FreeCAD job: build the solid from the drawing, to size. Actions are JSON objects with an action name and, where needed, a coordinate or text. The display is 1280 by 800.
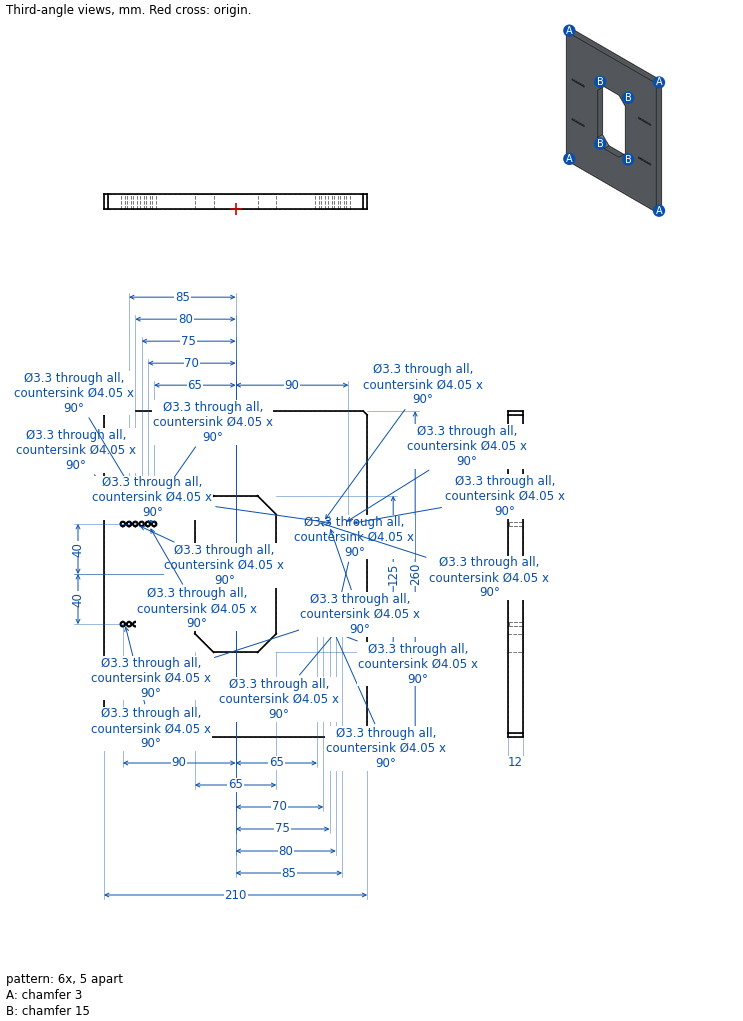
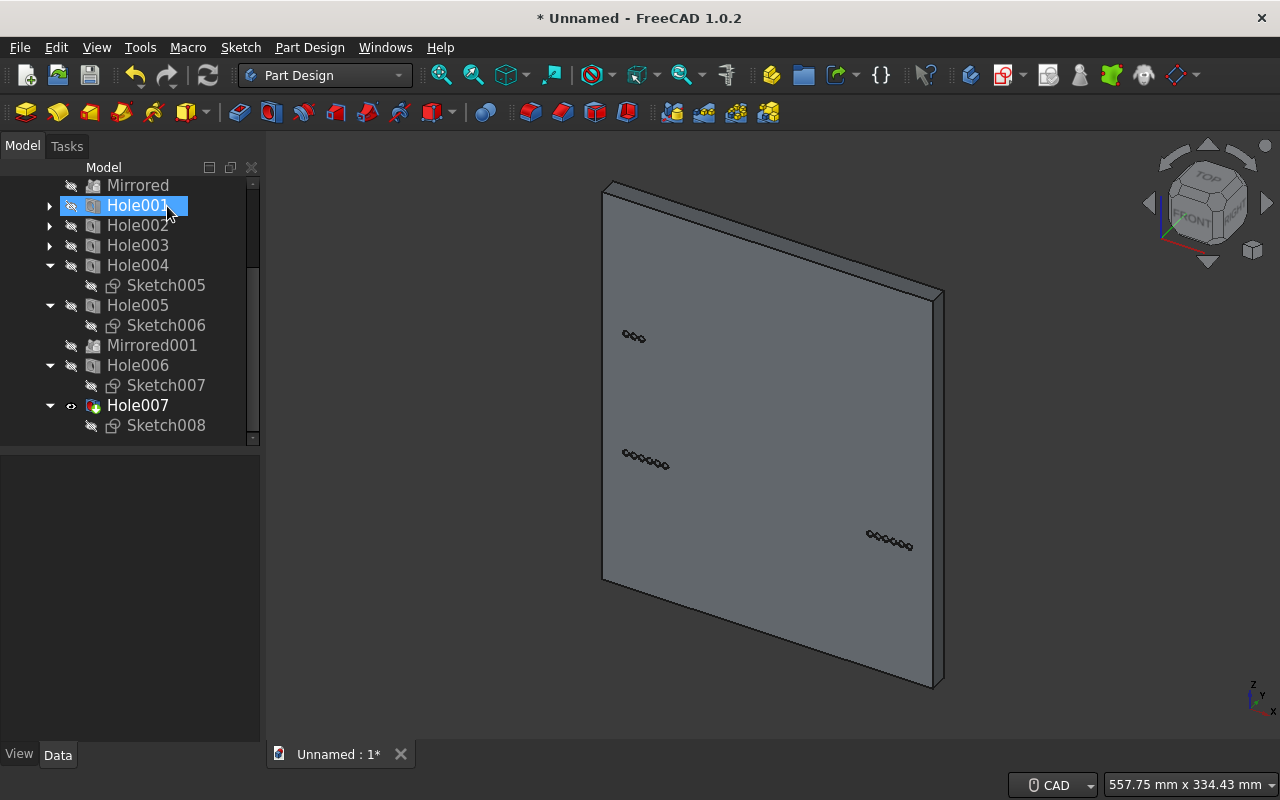
{"action": "left_click", "coordinate": [1004, 76]}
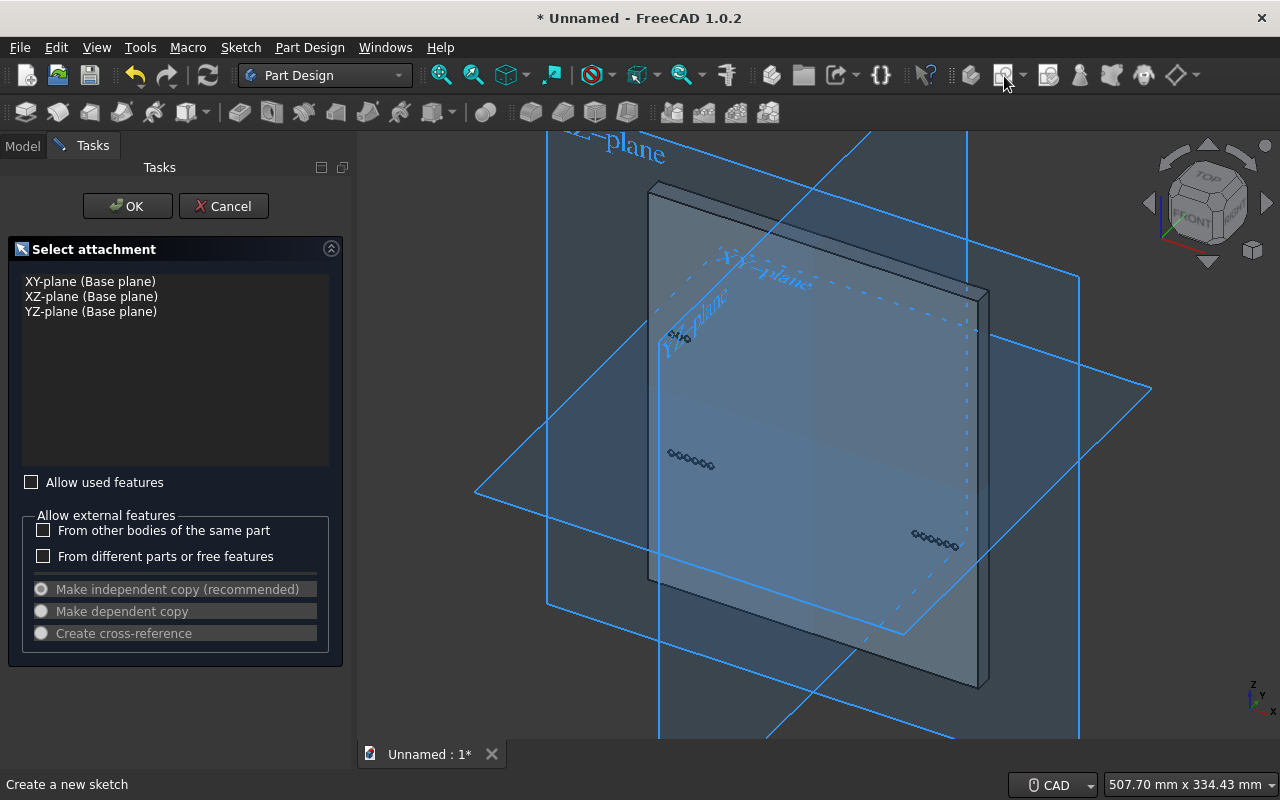
{"action": "left_click", "coordinate": [82, 296]}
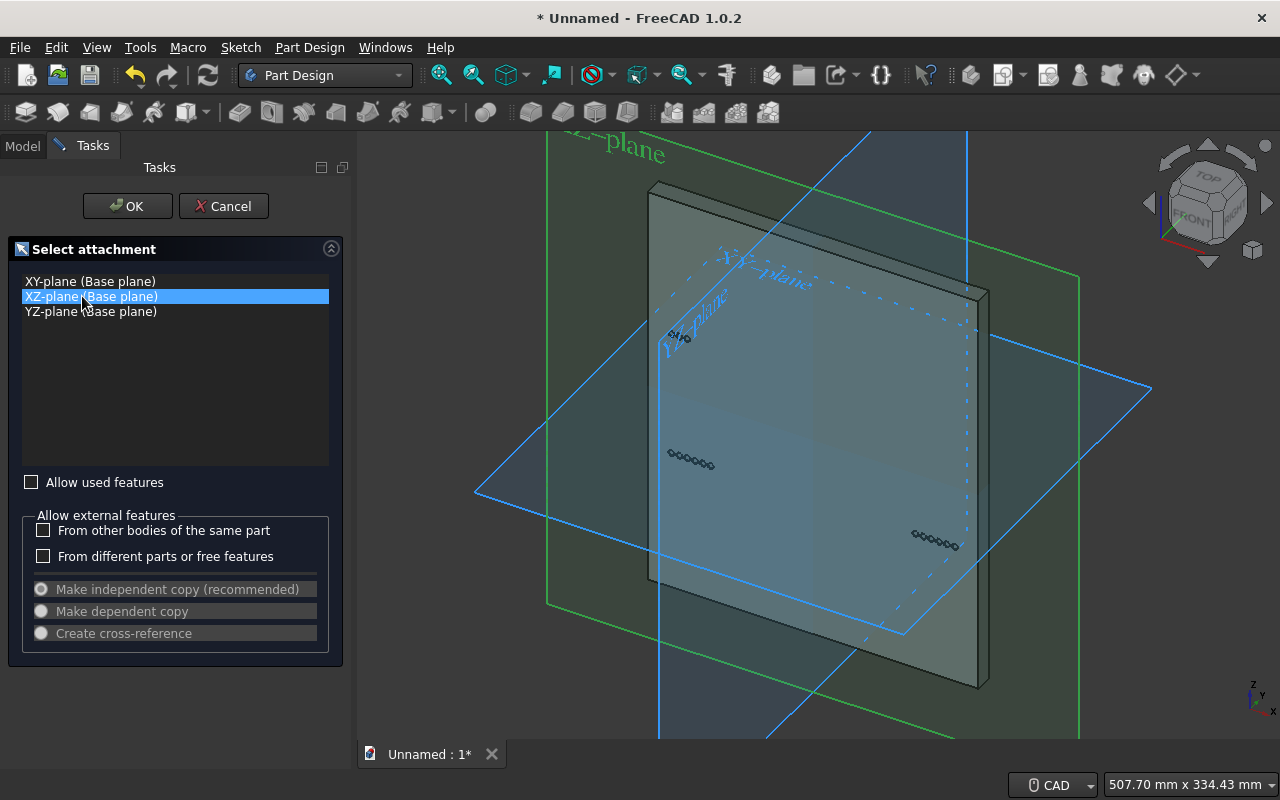
{"action": "left_click", "coordinate": [128, 206]}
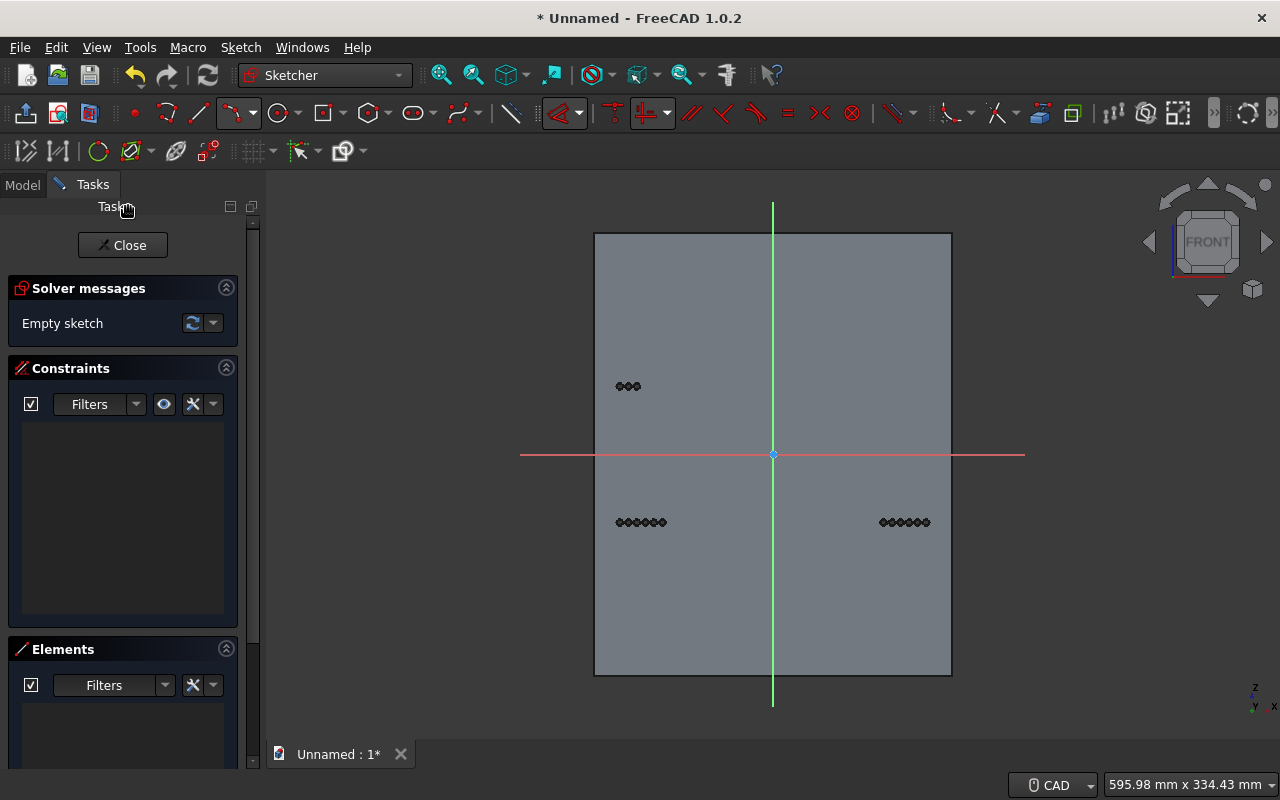
{"action": "scroll", "coordinate": [642, 383], "scroll_direction": "up", "scroll_amount": 15}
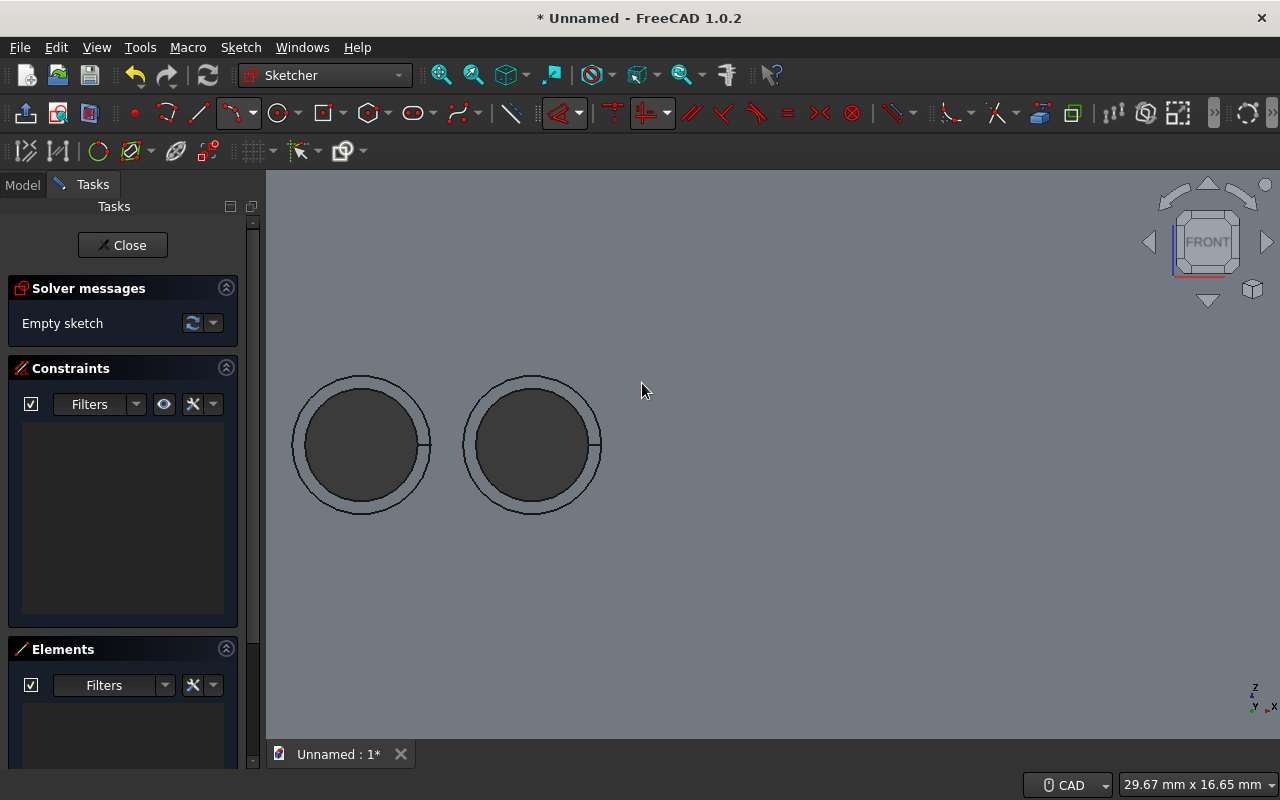
{"action": "scroll", "coordinate": [703, 441], "scroll_direction": "up", "scroll_amount": 6}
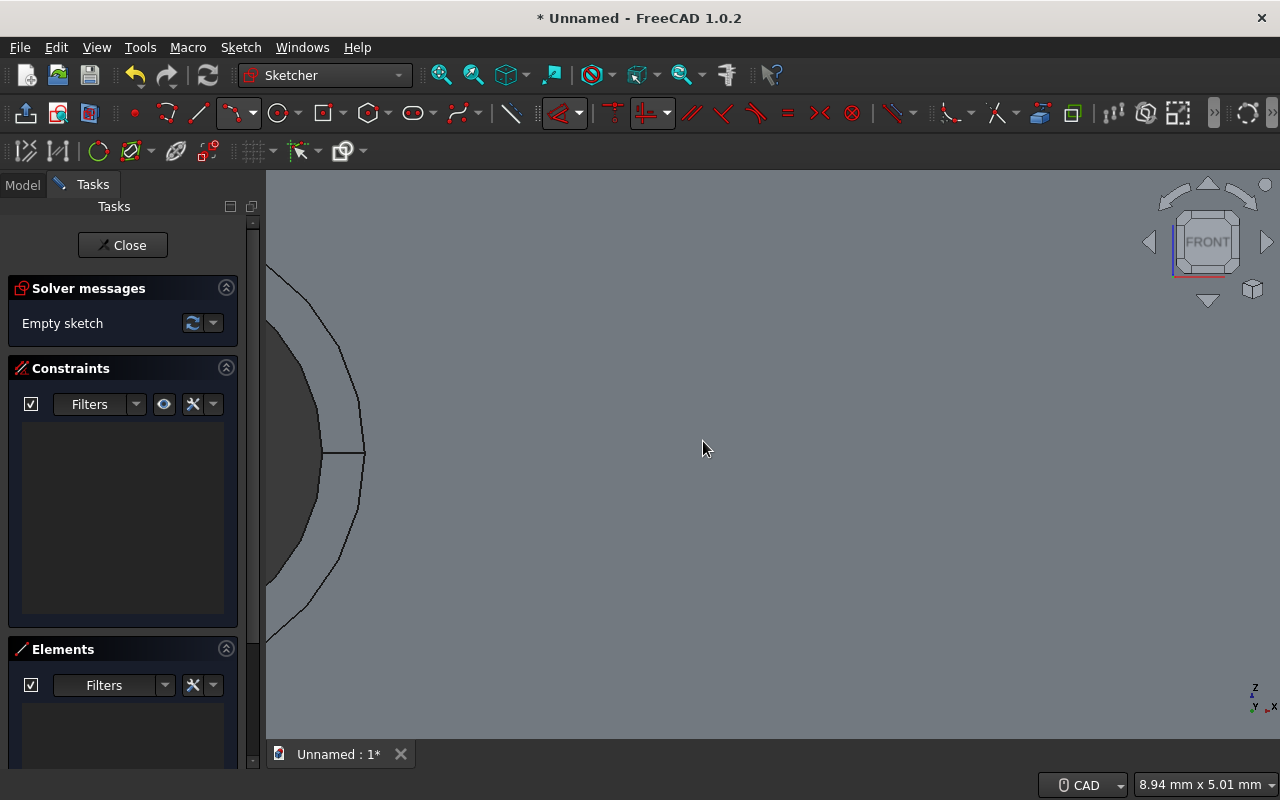
{"action": "left_click", "coordinate": [278, 114]}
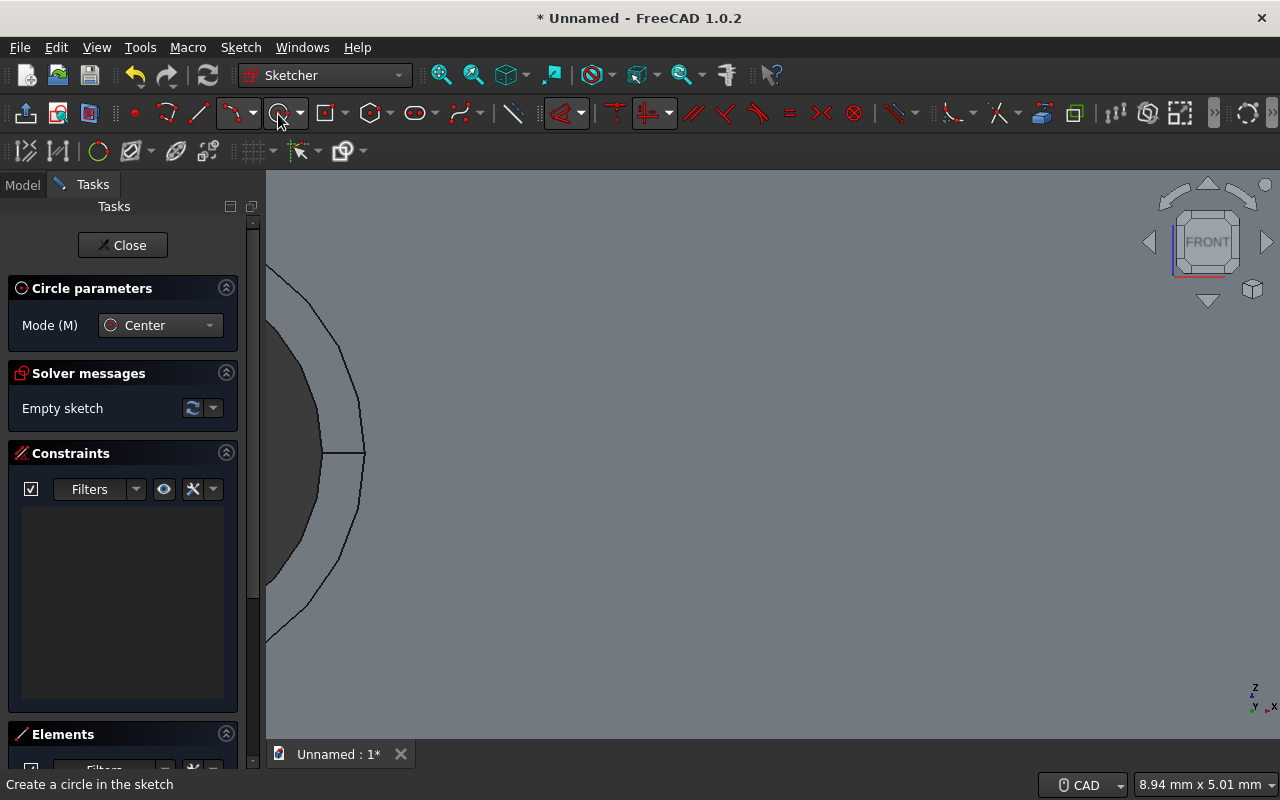
{"action": "left_click", "coordinate": [702, 453]}
{"action": "mouse_move", "coordinate": [835, 321]}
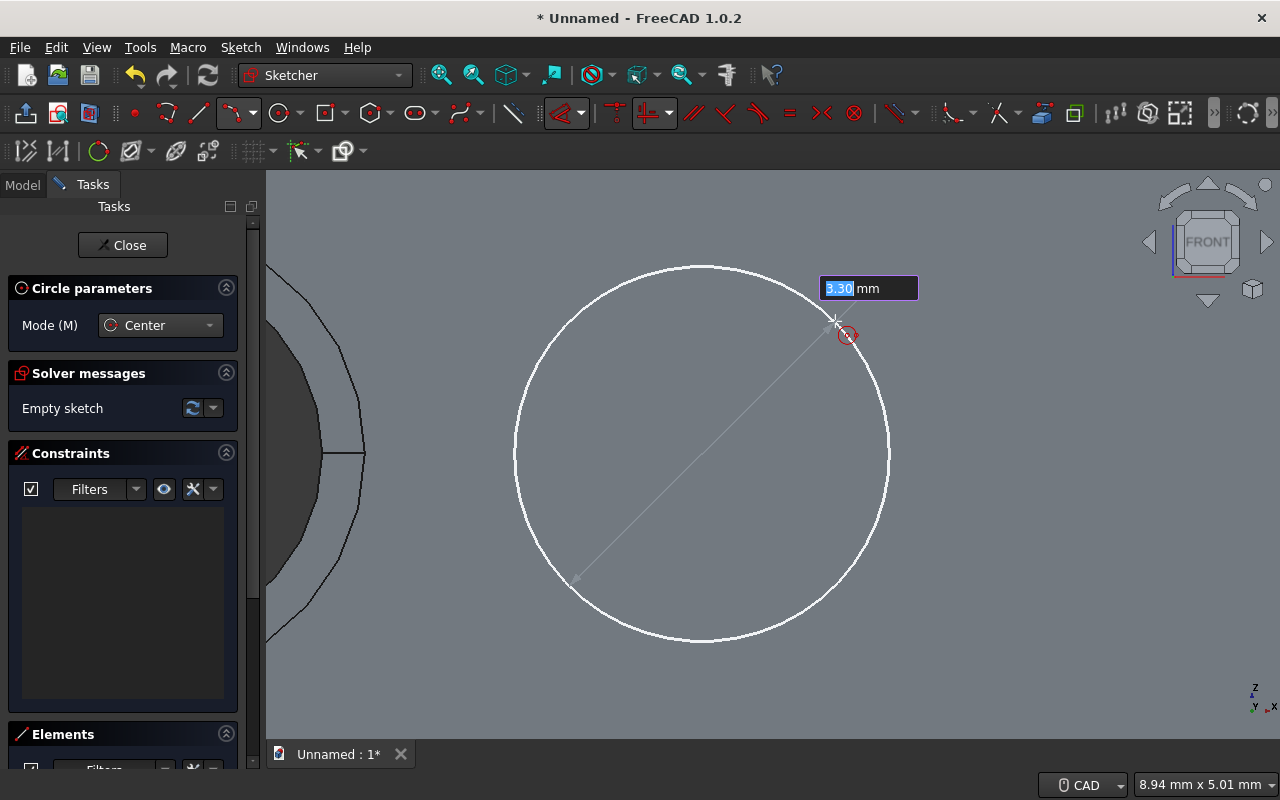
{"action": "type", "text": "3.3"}
{"action": "key", "text": "Return"}
{"action": "key", "text": "Escape"}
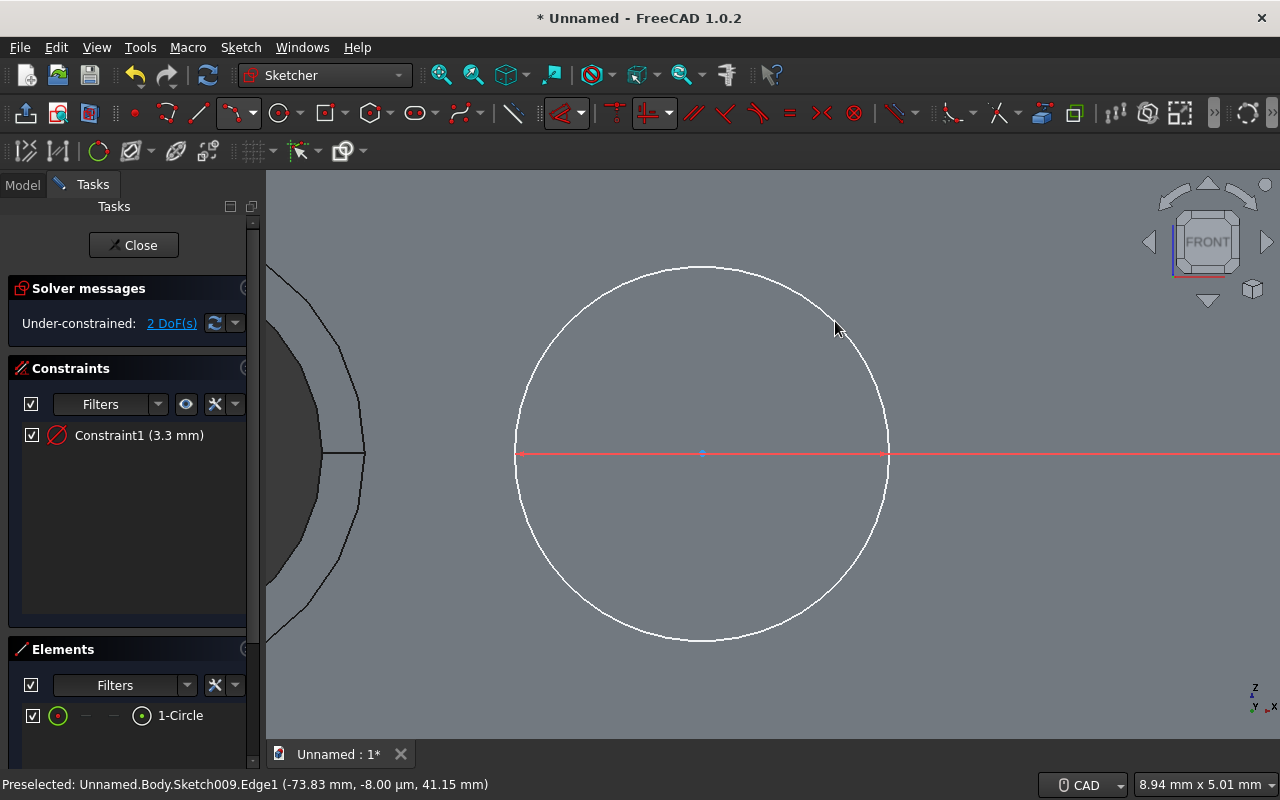
{"action": "left_click", "coordinate": [702, 454]}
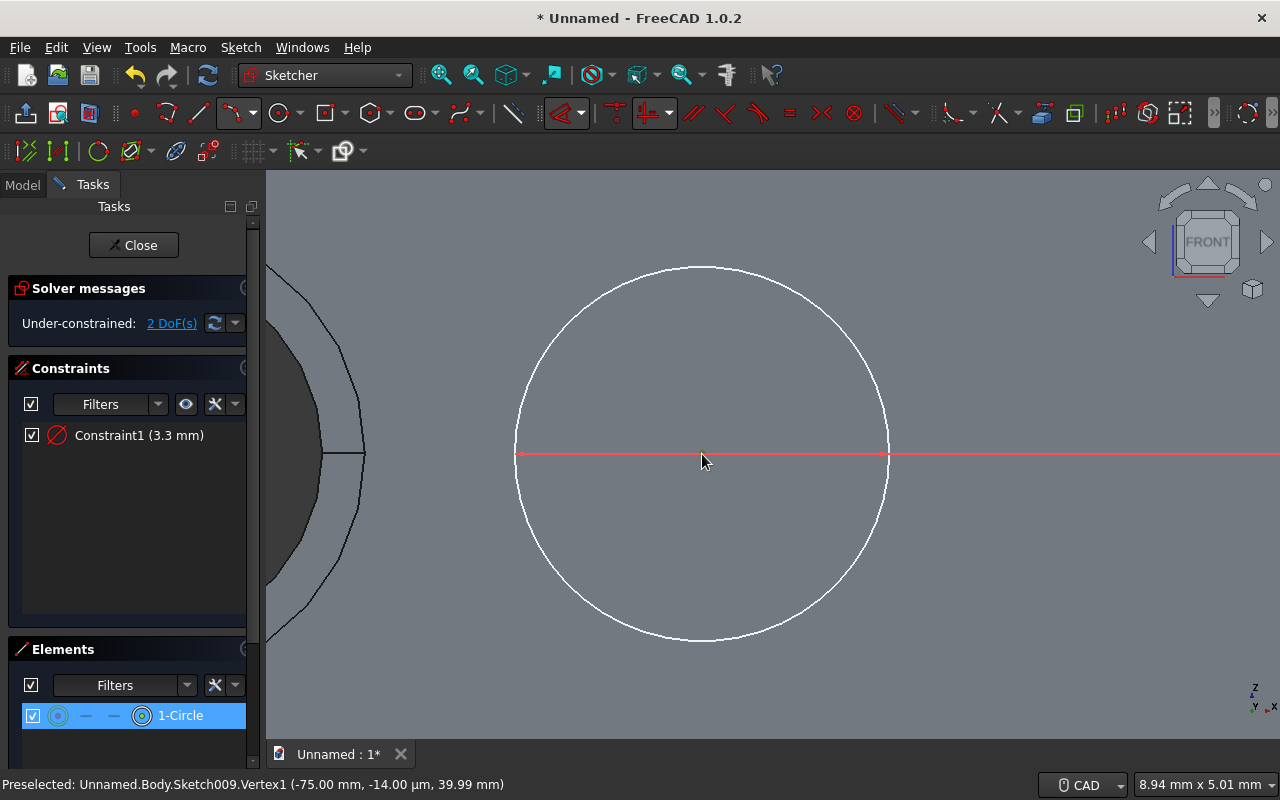
{"action": "key", "text": "l"}